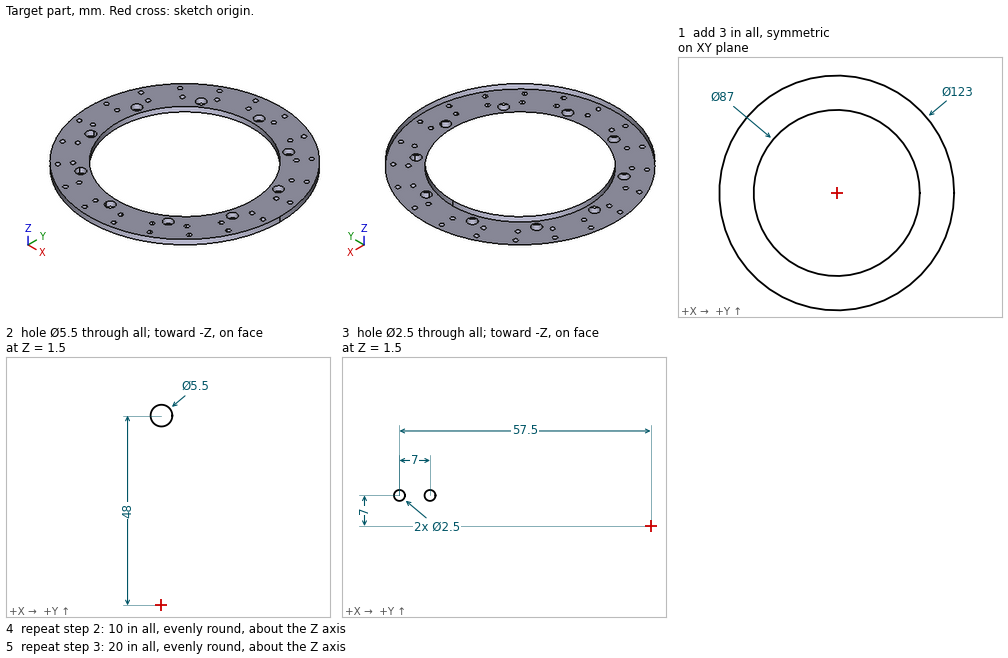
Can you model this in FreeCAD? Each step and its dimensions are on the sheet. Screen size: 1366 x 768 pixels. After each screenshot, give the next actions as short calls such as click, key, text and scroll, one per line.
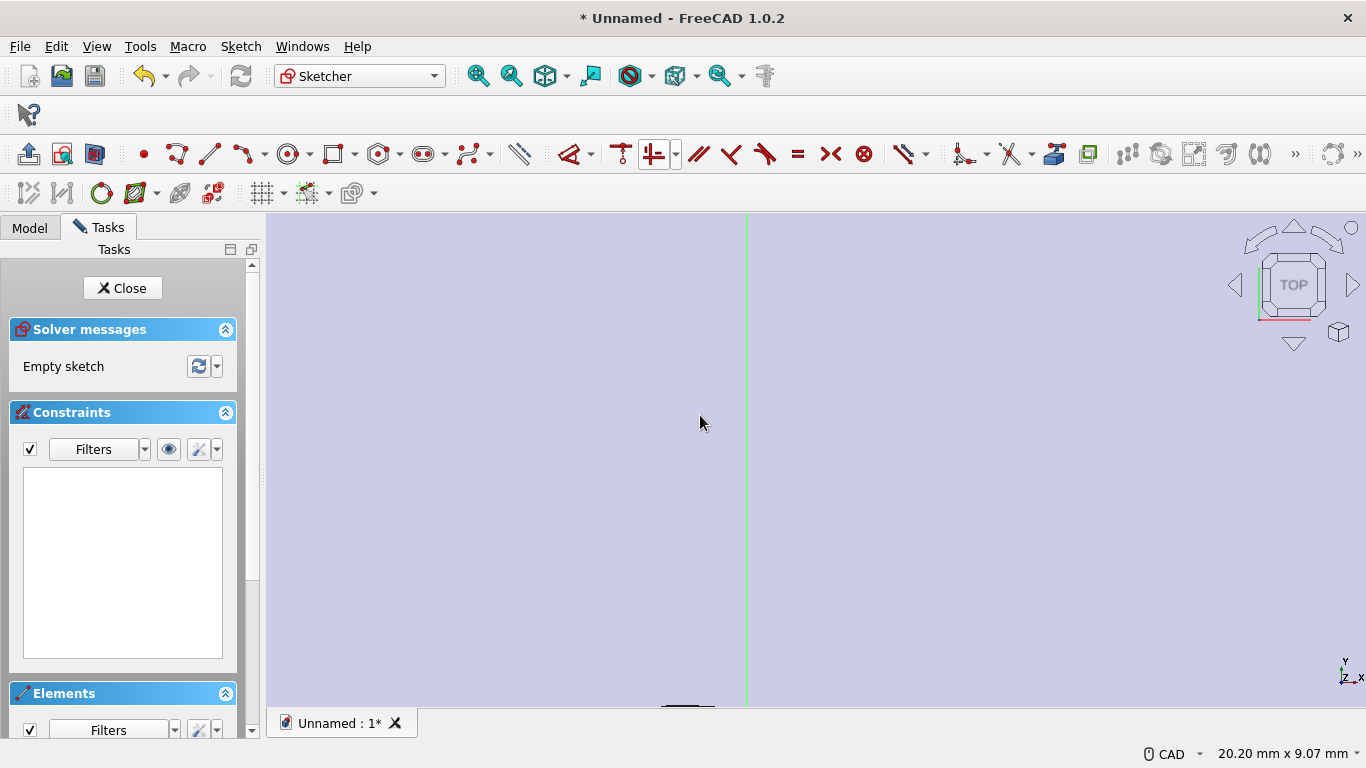
key(g)
key(c)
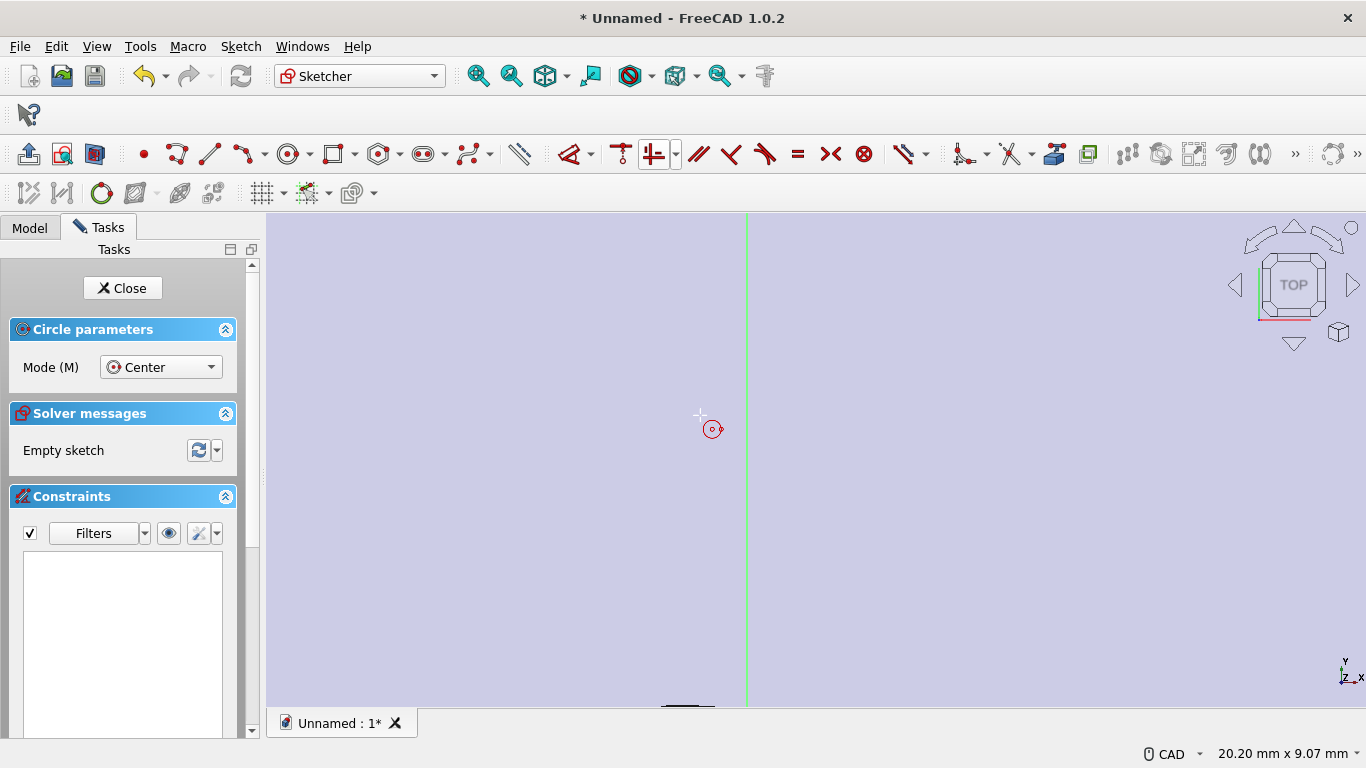
click(747, 460)
move(853, 354)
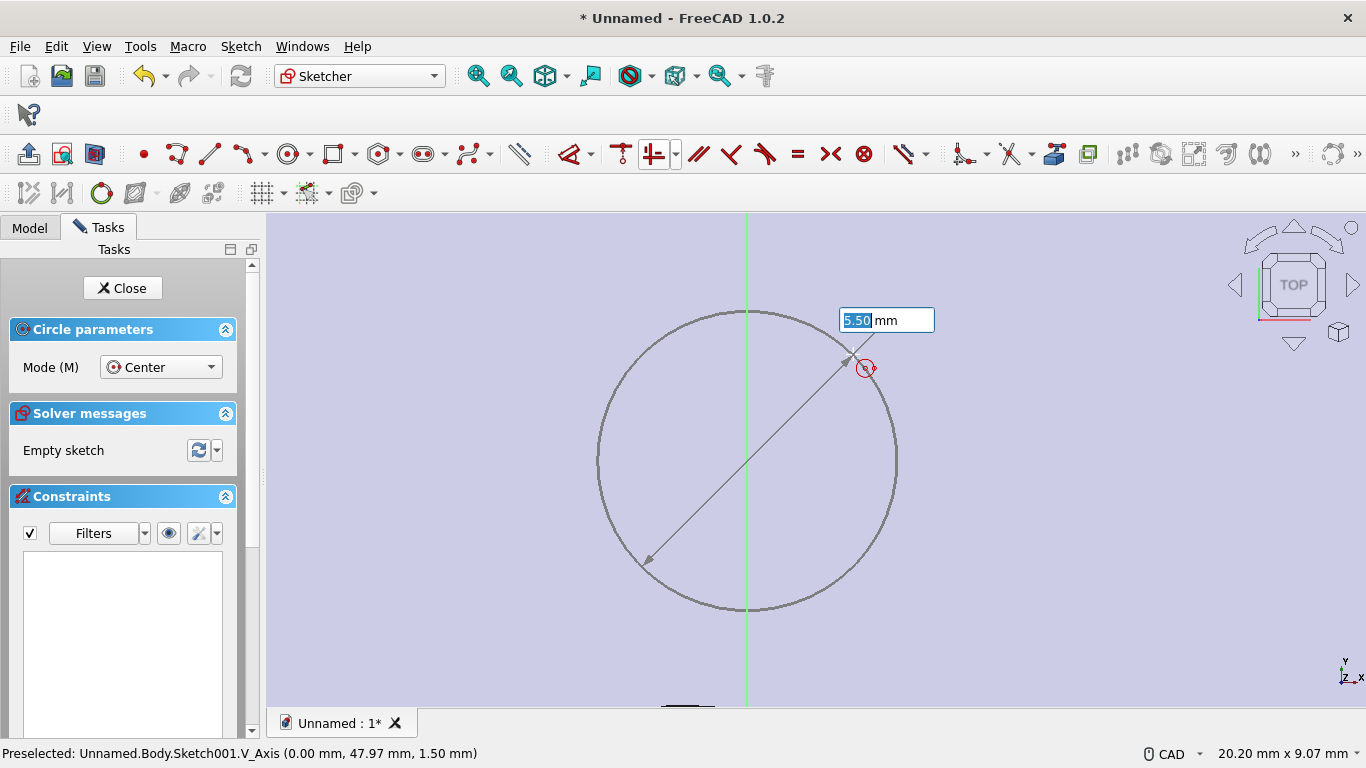
text(5.5)
key(Return)
key(Escape)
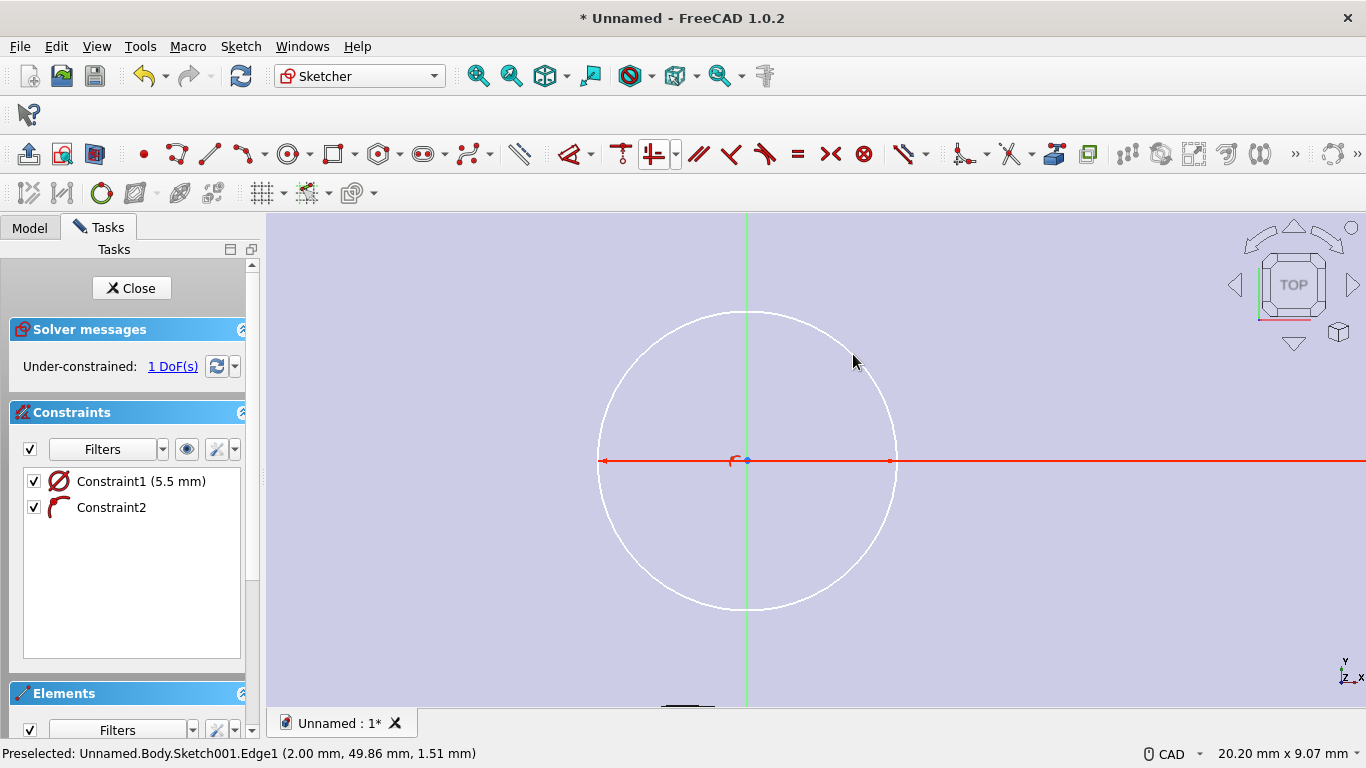
click(747, 461)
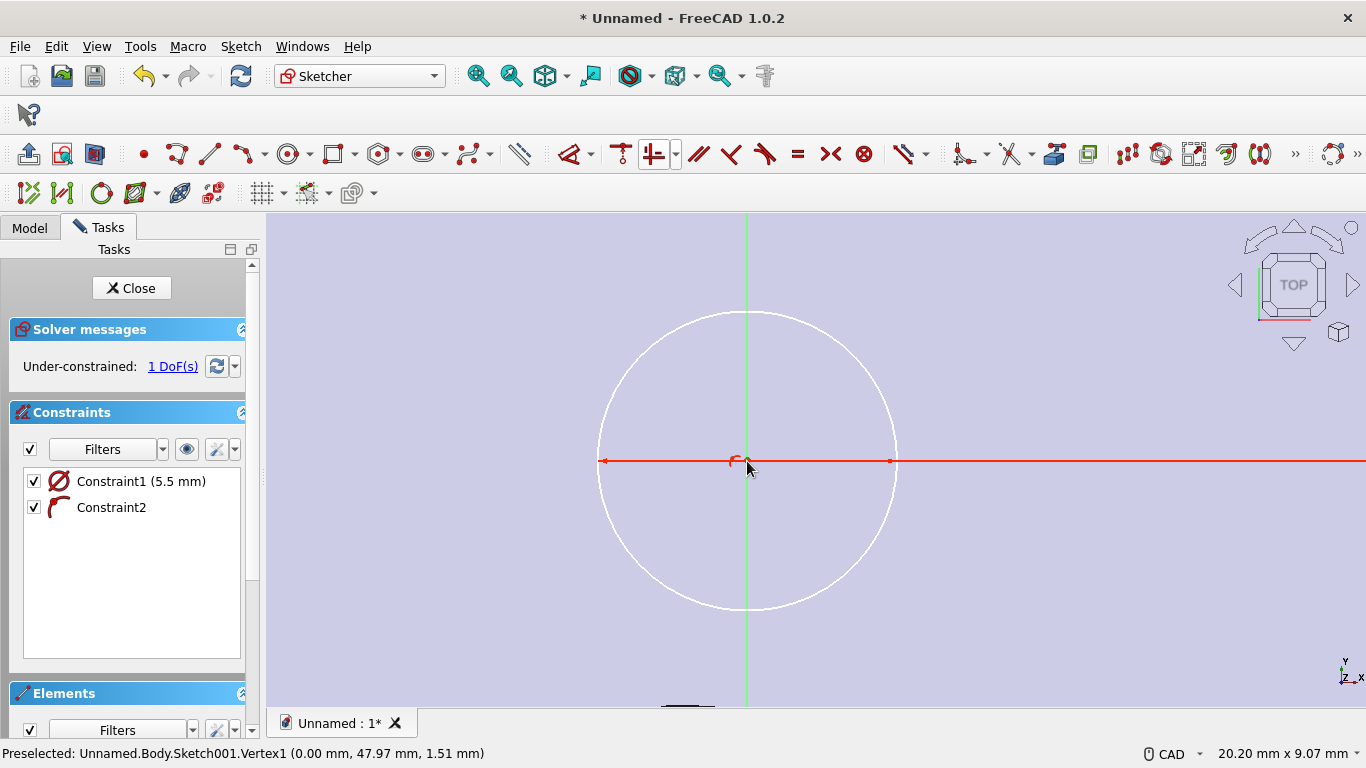
click(590, 154)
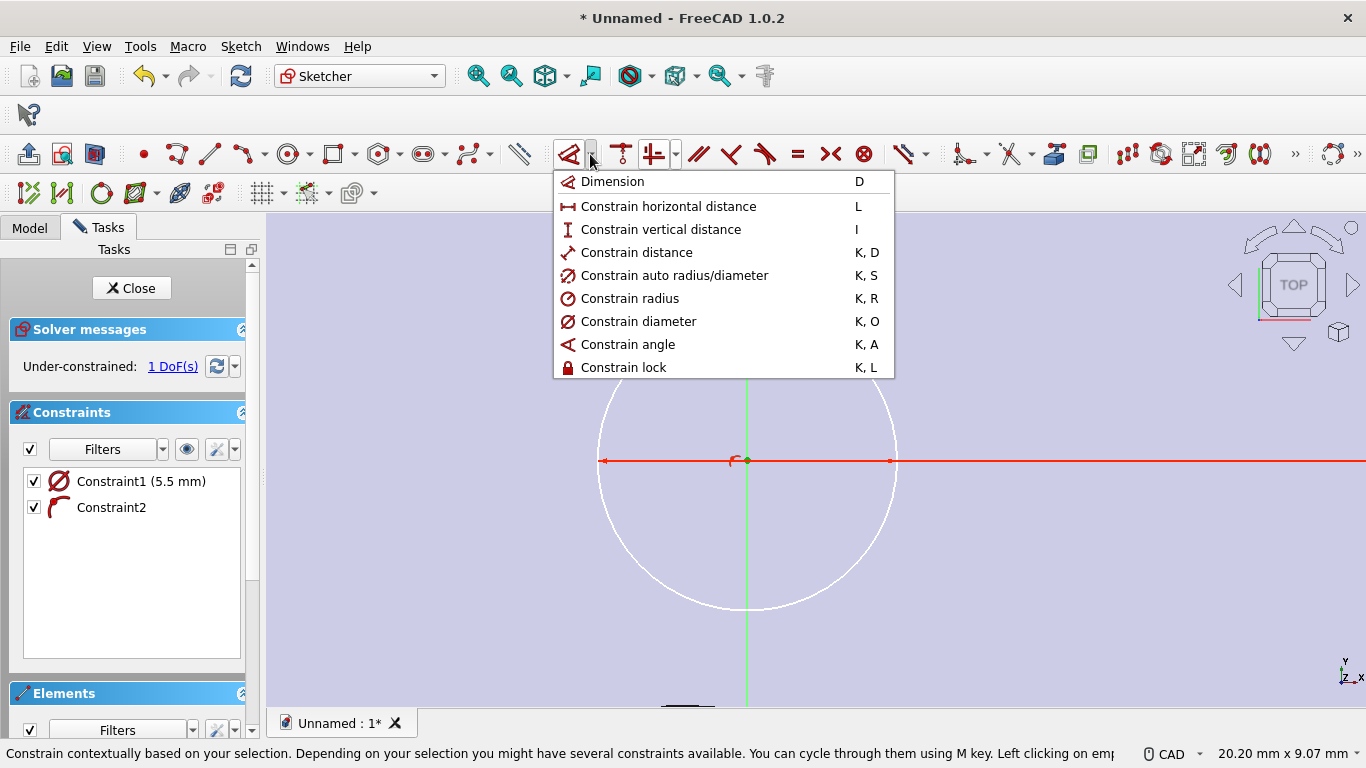
click(724, 230)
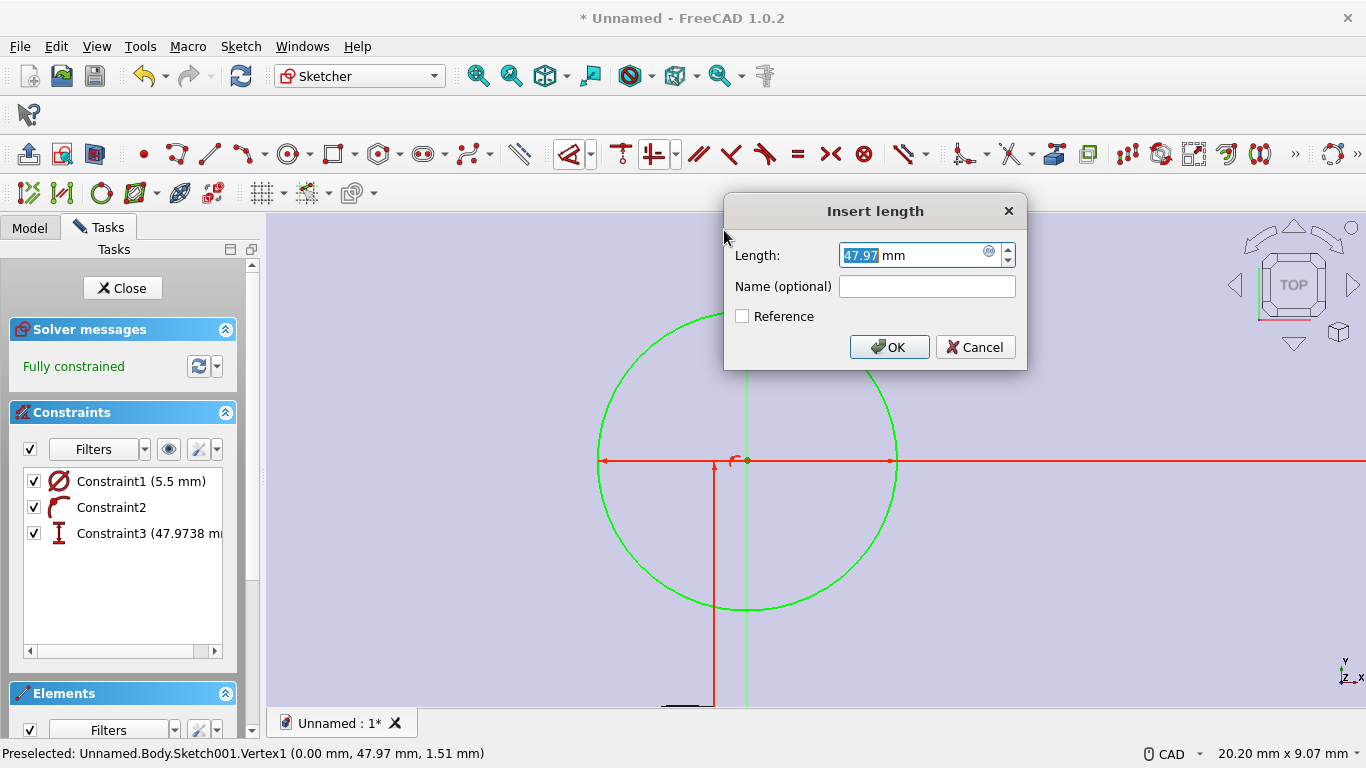
text(48)
key(Return)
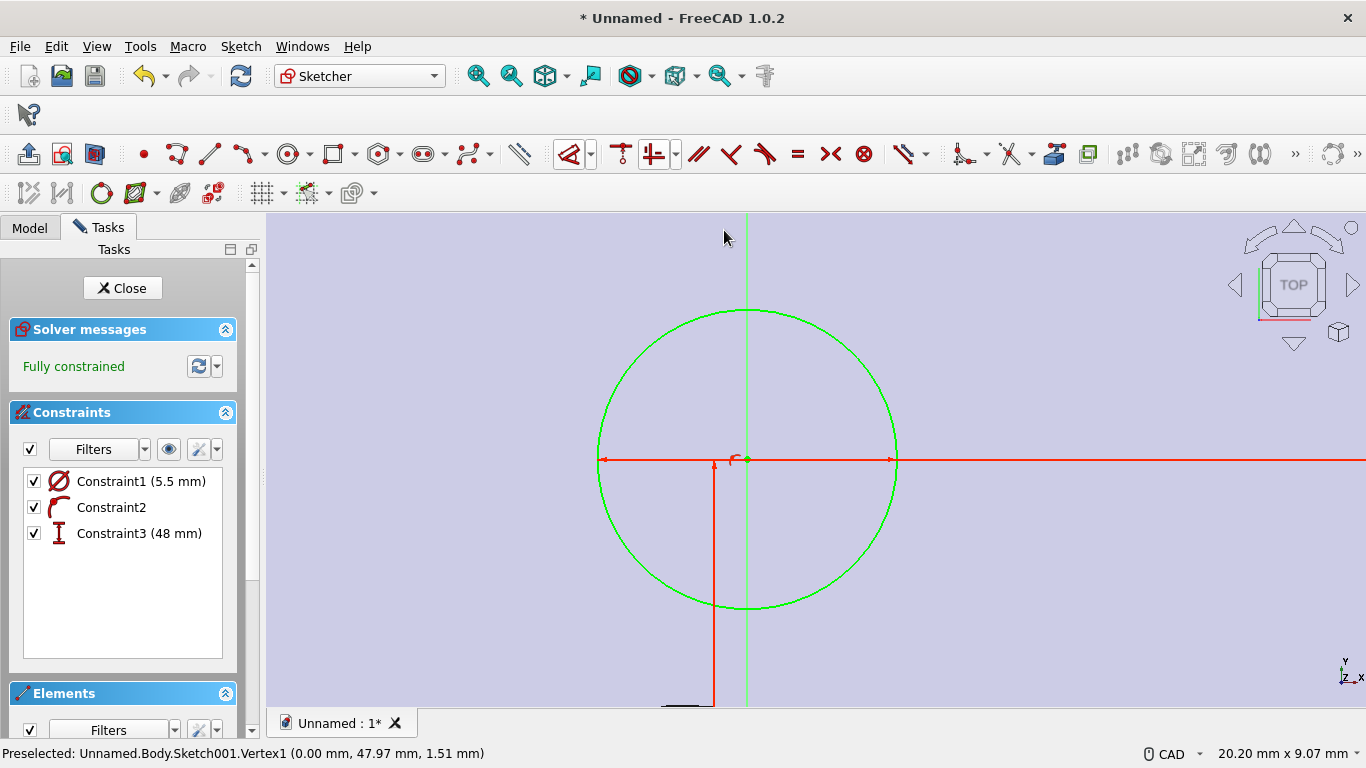
click(123, 288)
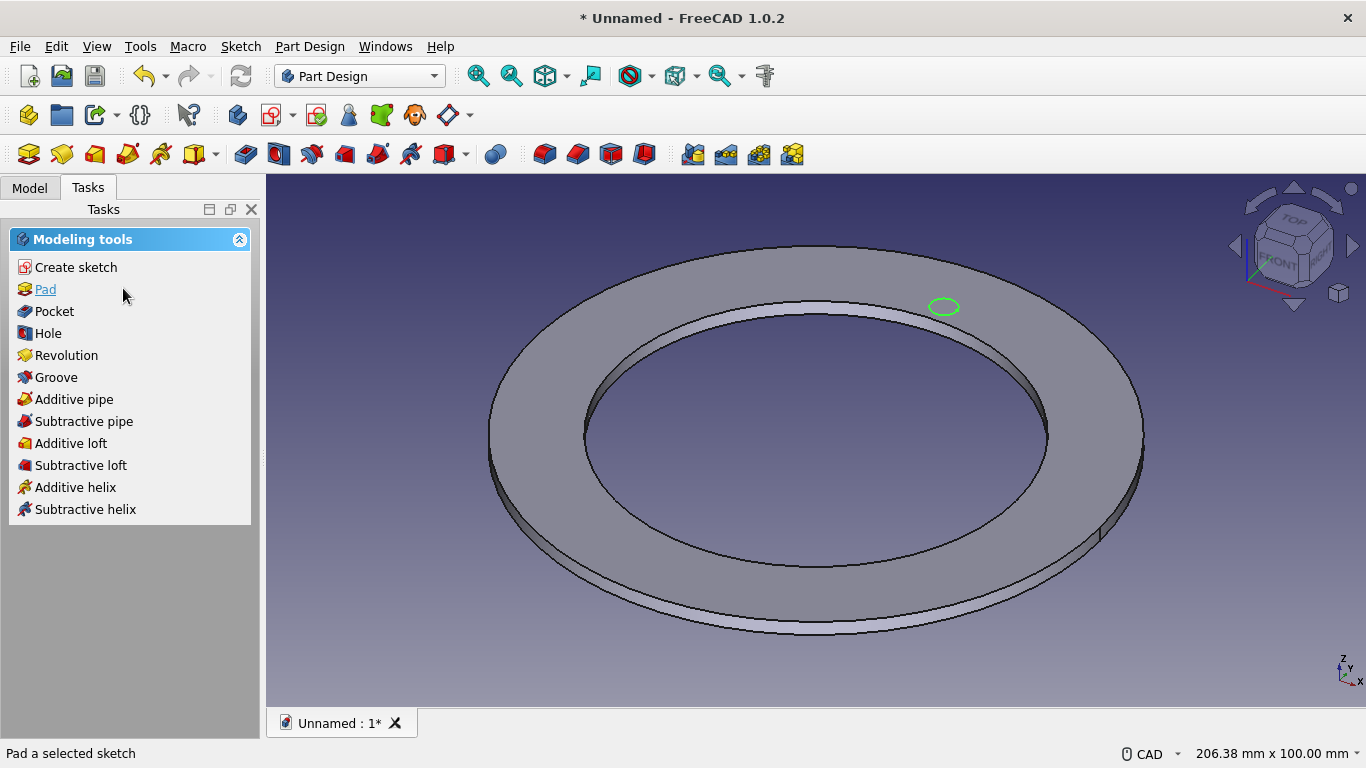
click(279, 154)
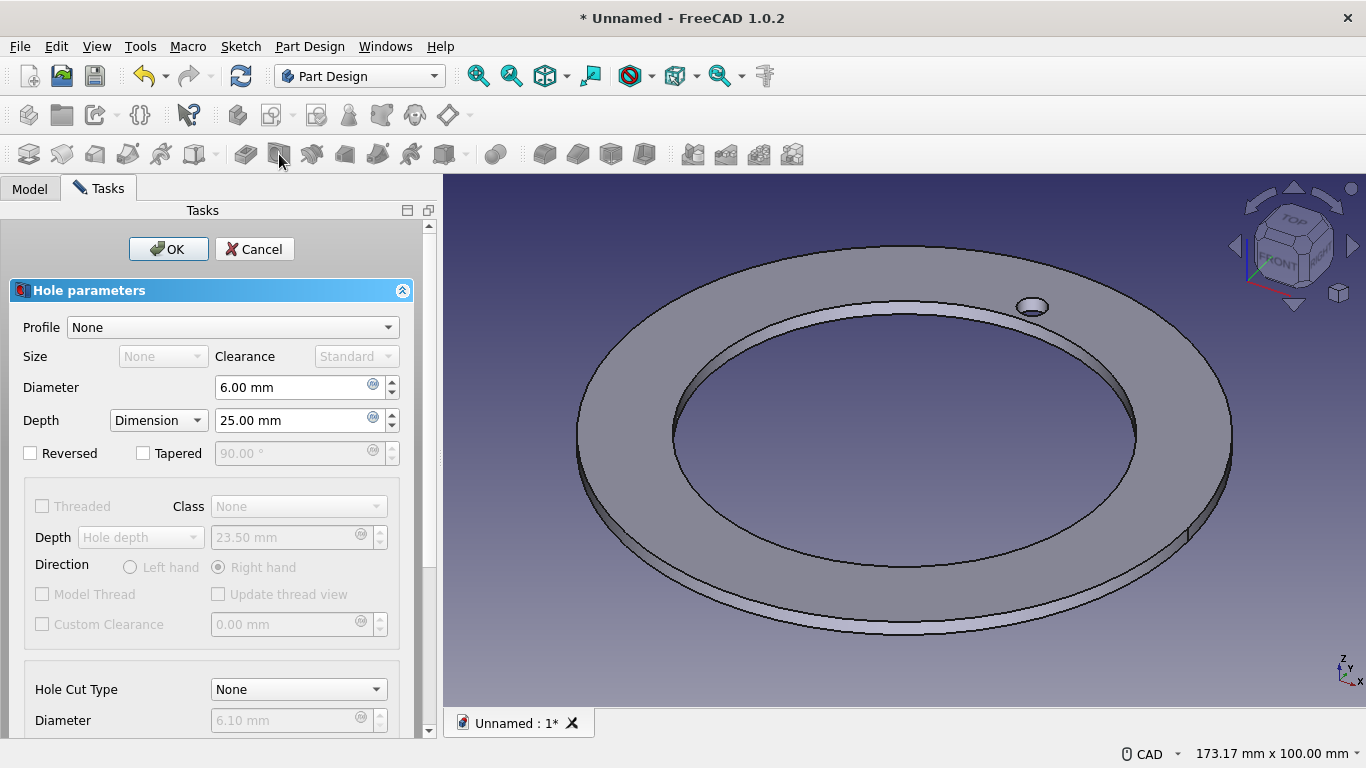
triple_click(300, 388)